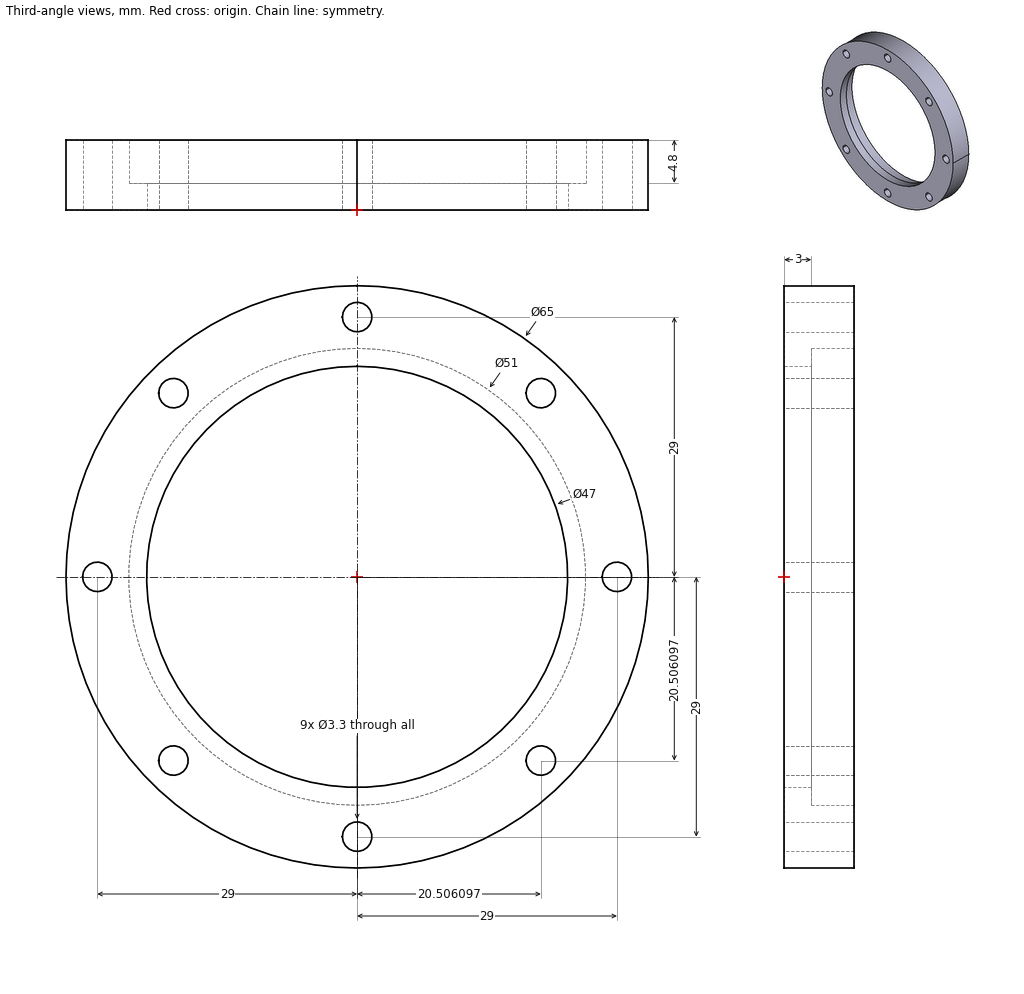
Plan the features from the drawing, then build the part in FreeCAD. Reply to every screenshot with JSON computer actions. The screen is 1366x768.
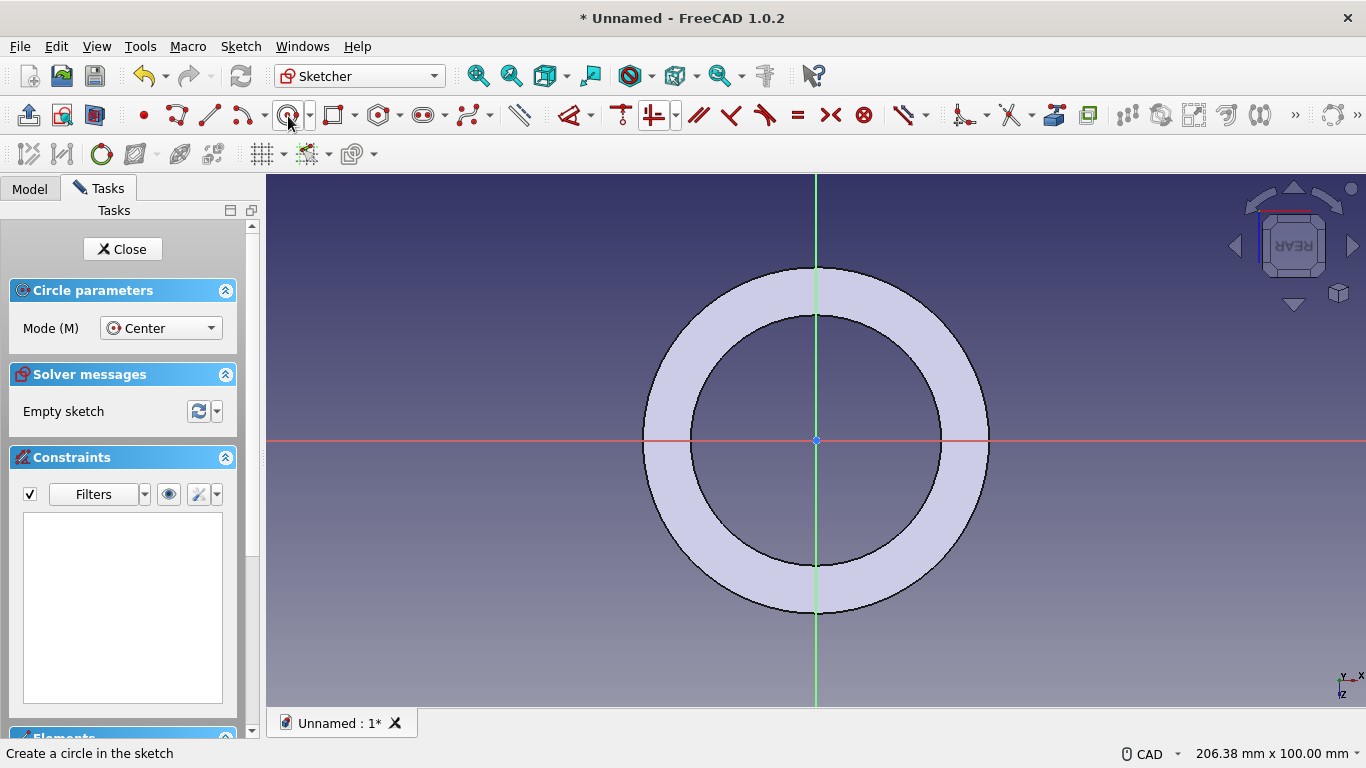
{"action": "left_click", "coordinate": [816, 441]}
{"action": "mouse_move", "coordinate": [938, 318]}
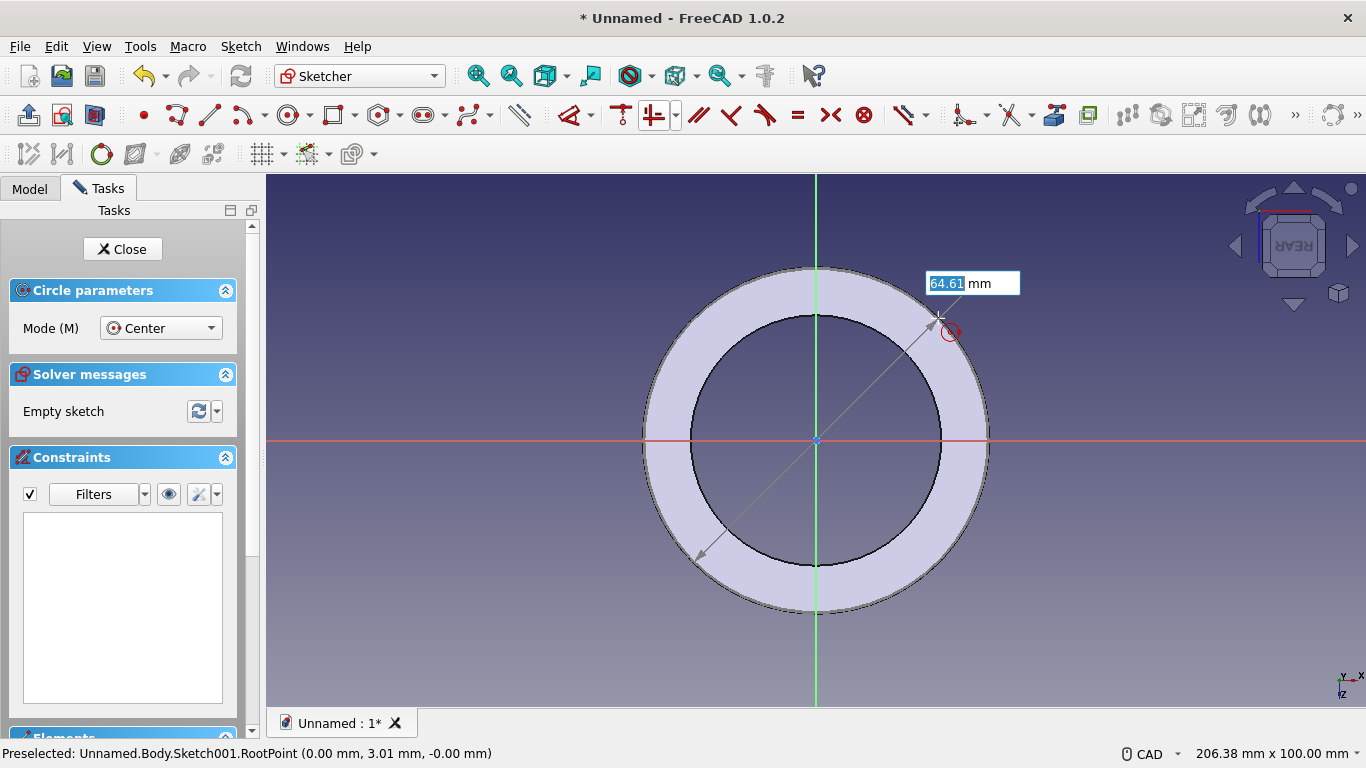
{"action": "type", "text": "65"}
{"action": "key", "text": "Return"}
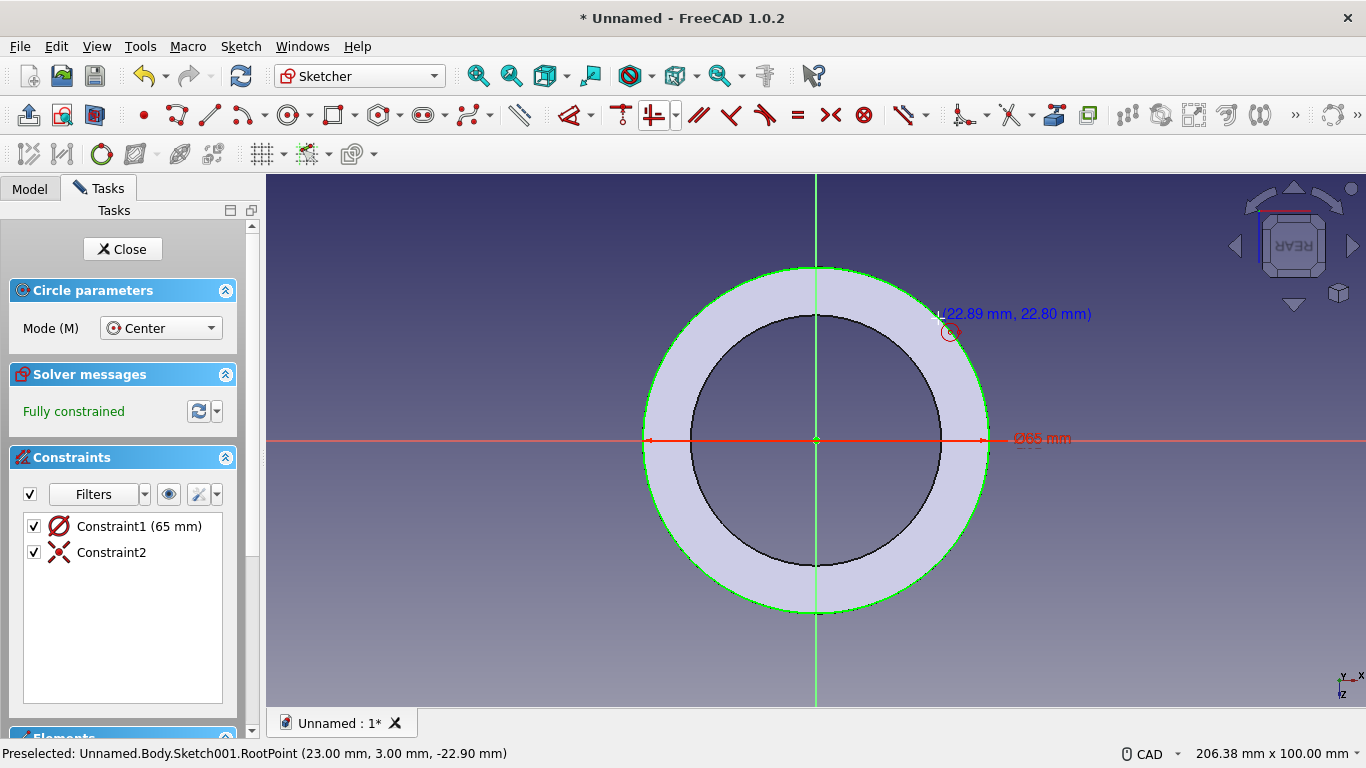
{"action": "left_click", "coordinate": [816, 441]}
{"action": "mouse_move", "coordinate": [912, 344]}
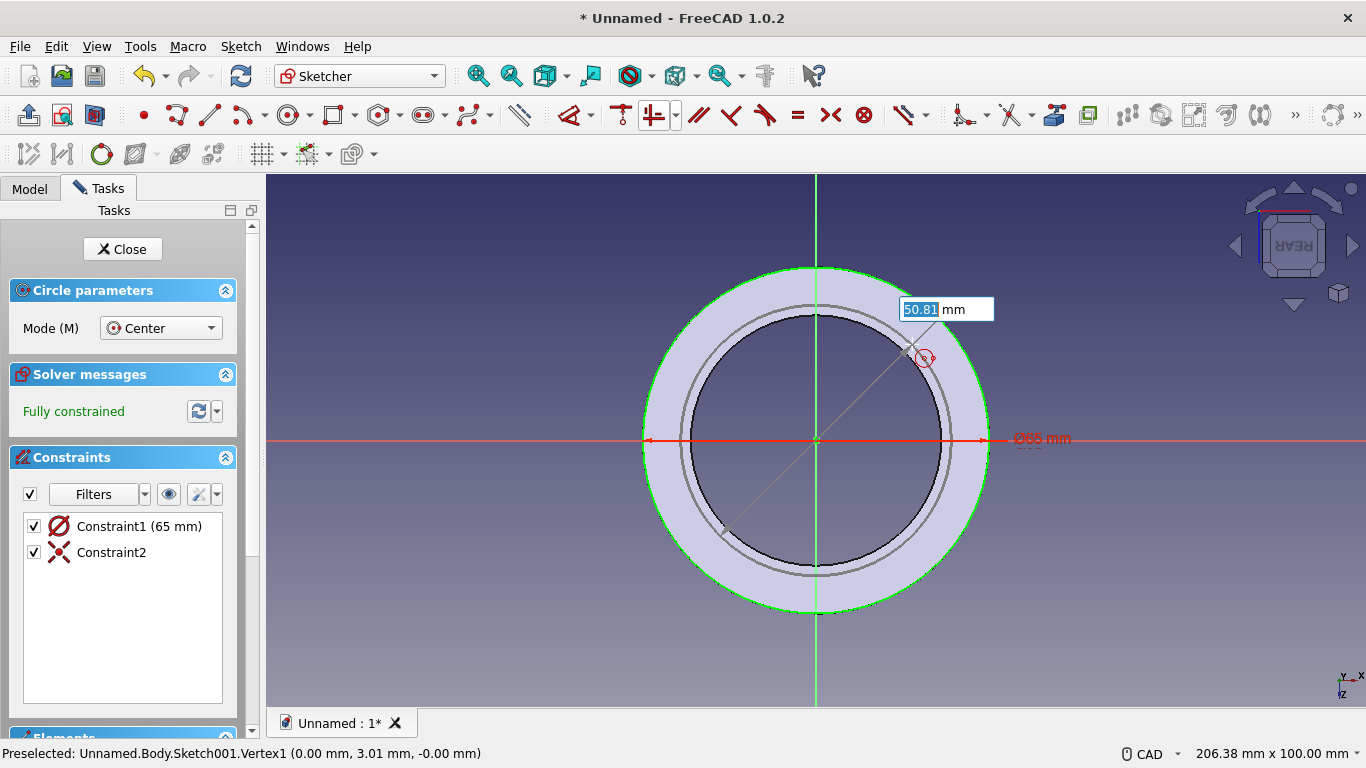
{"action": "type", "text": "51"}
{"action": "key", "text": "Return"}
{"action": "key", "text": "Escape"}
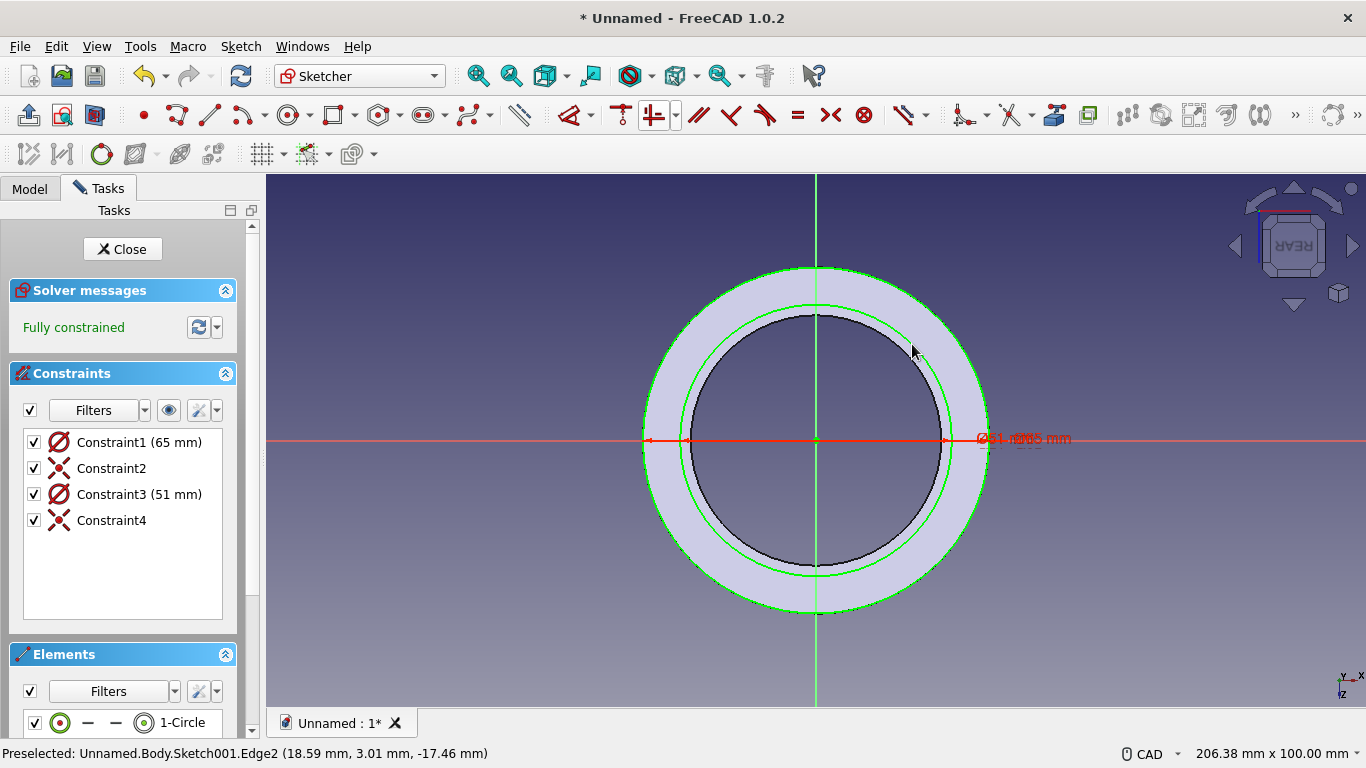
{"action": "left_click", "coordinate": [123, 249]}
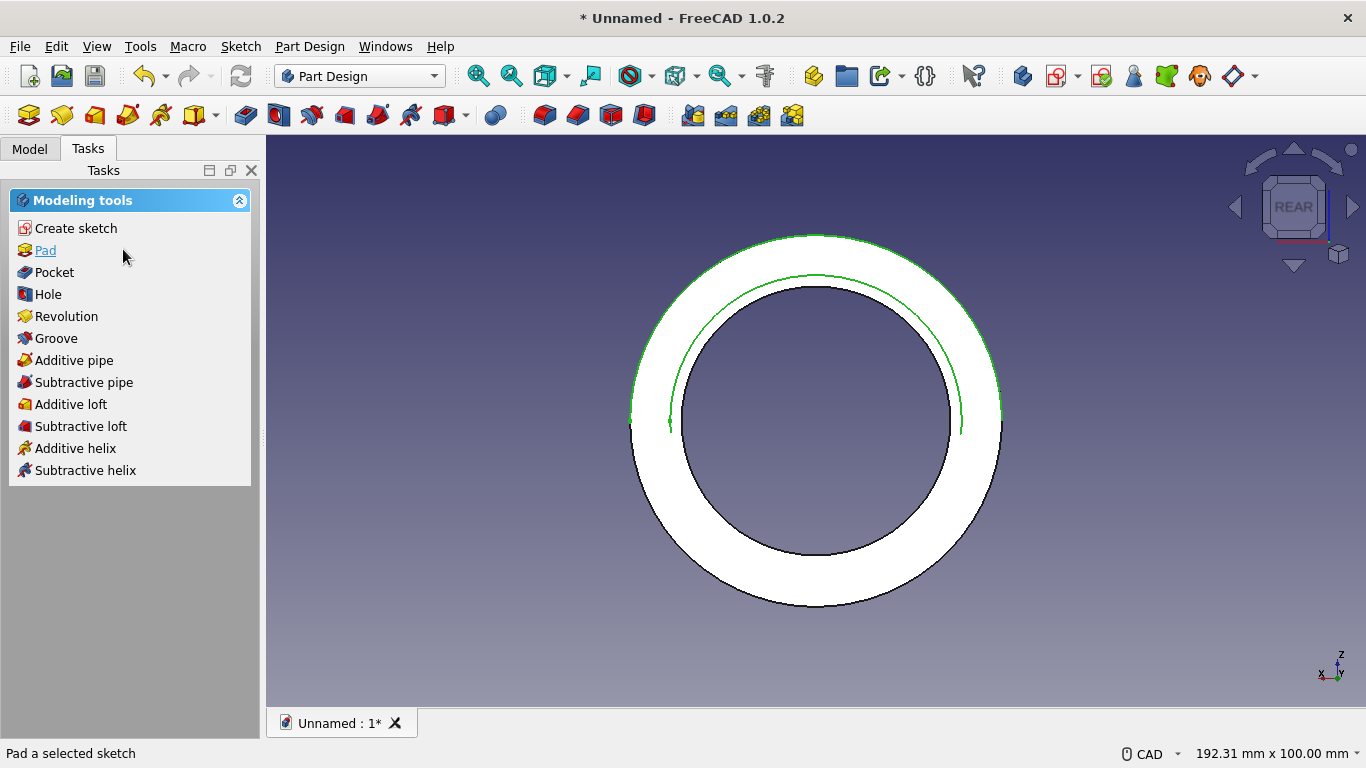
{"action": "left_click", "coordinate": [29, 116]}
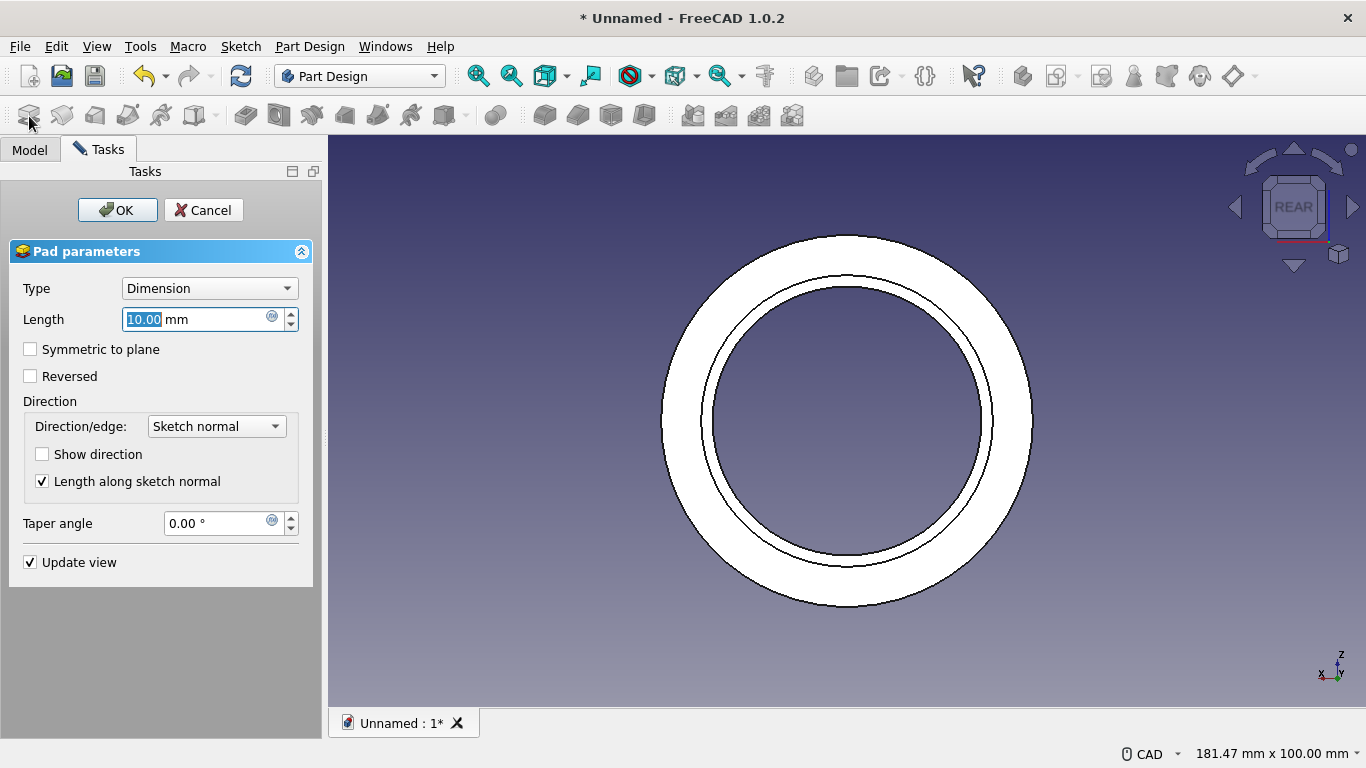
{"action": "type", "text": "4.8"}
{"action": "key", "text": "Tab"}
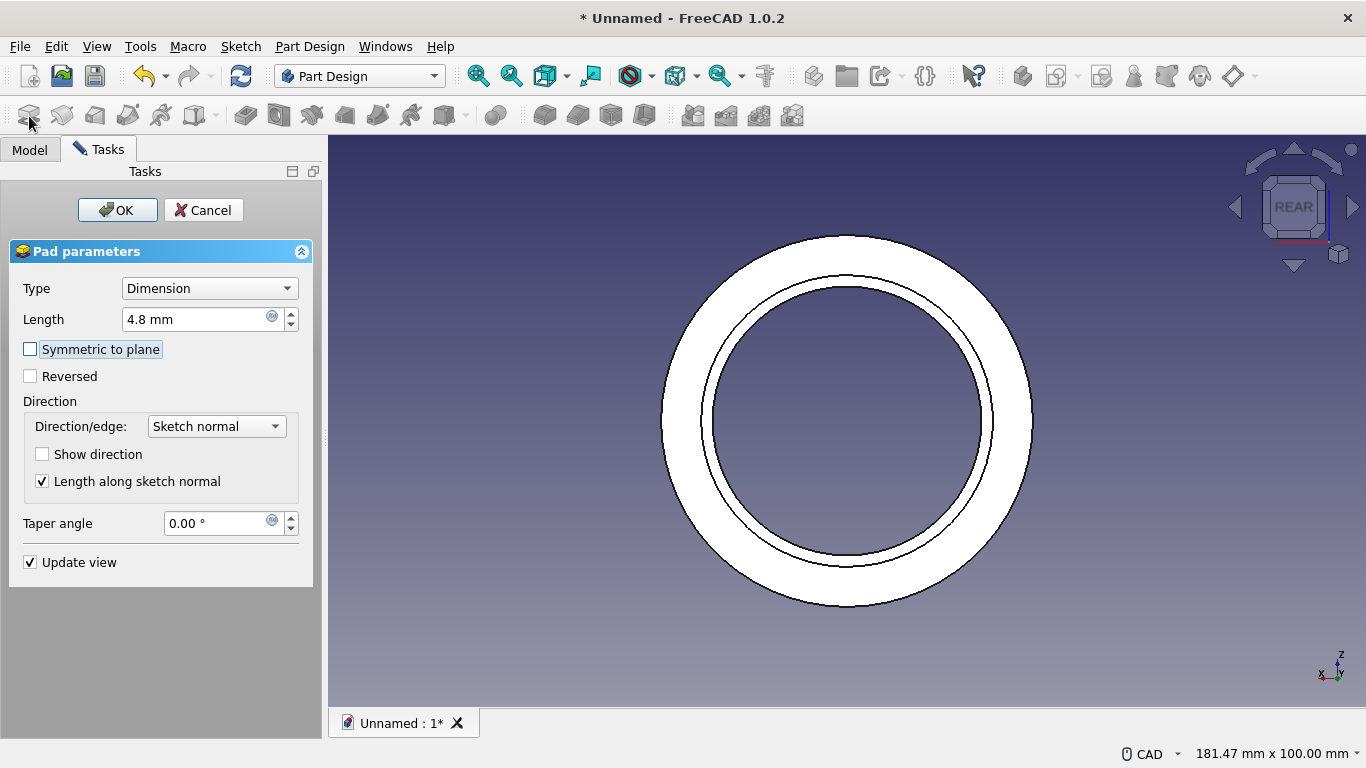
{"action": "left_click", "coordinate": [118, 210]}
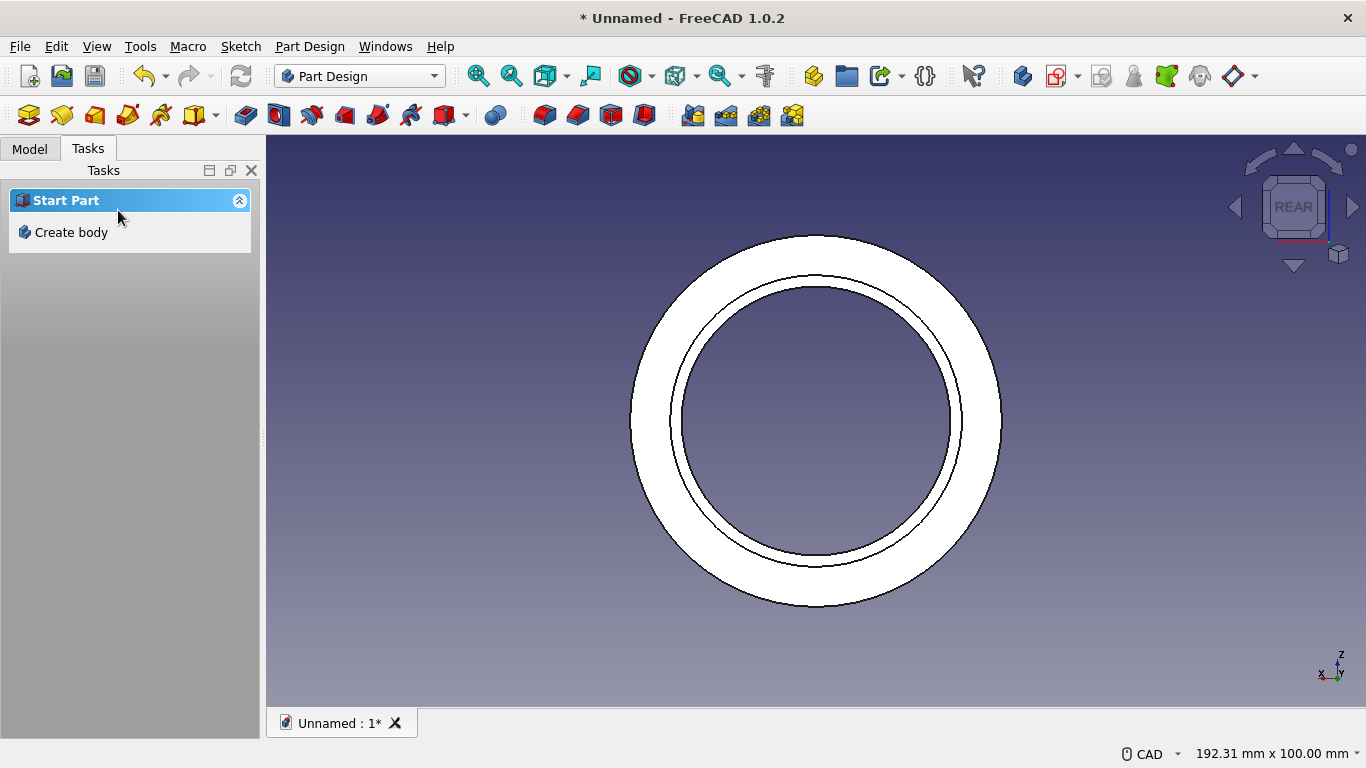
{"action": "left_click", "coordinate": [657, 367]}